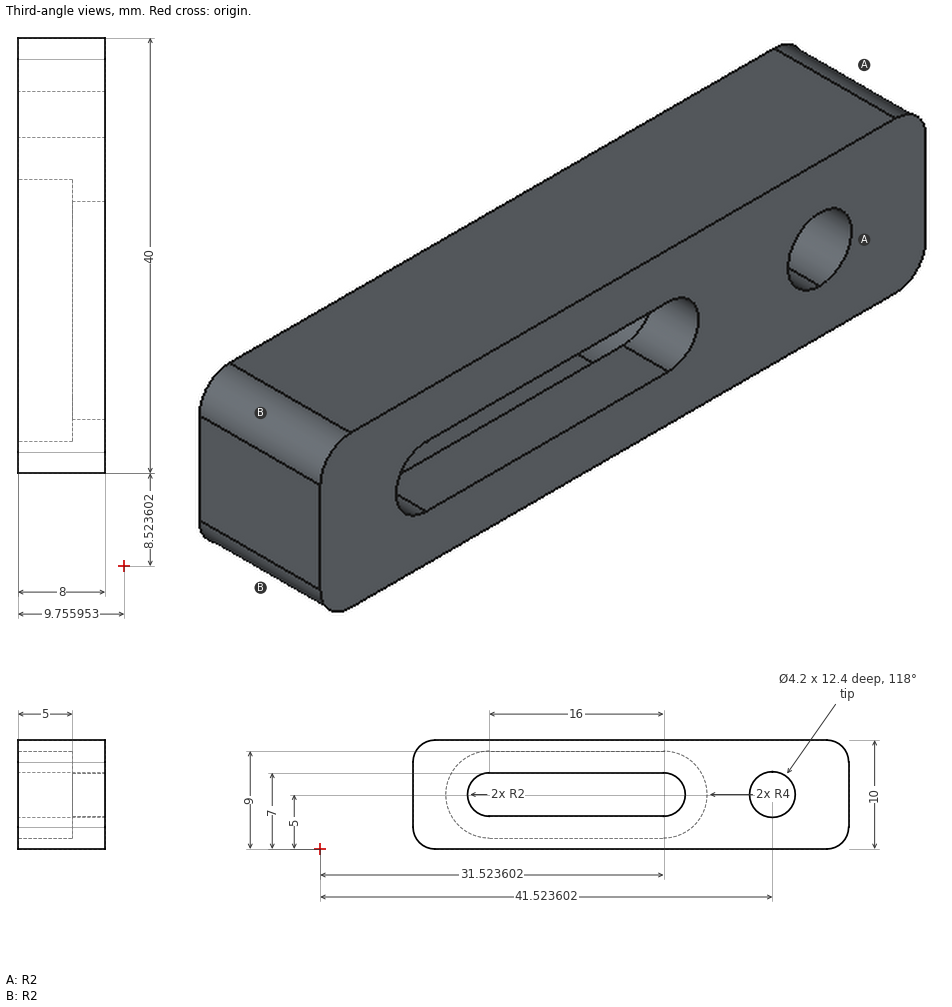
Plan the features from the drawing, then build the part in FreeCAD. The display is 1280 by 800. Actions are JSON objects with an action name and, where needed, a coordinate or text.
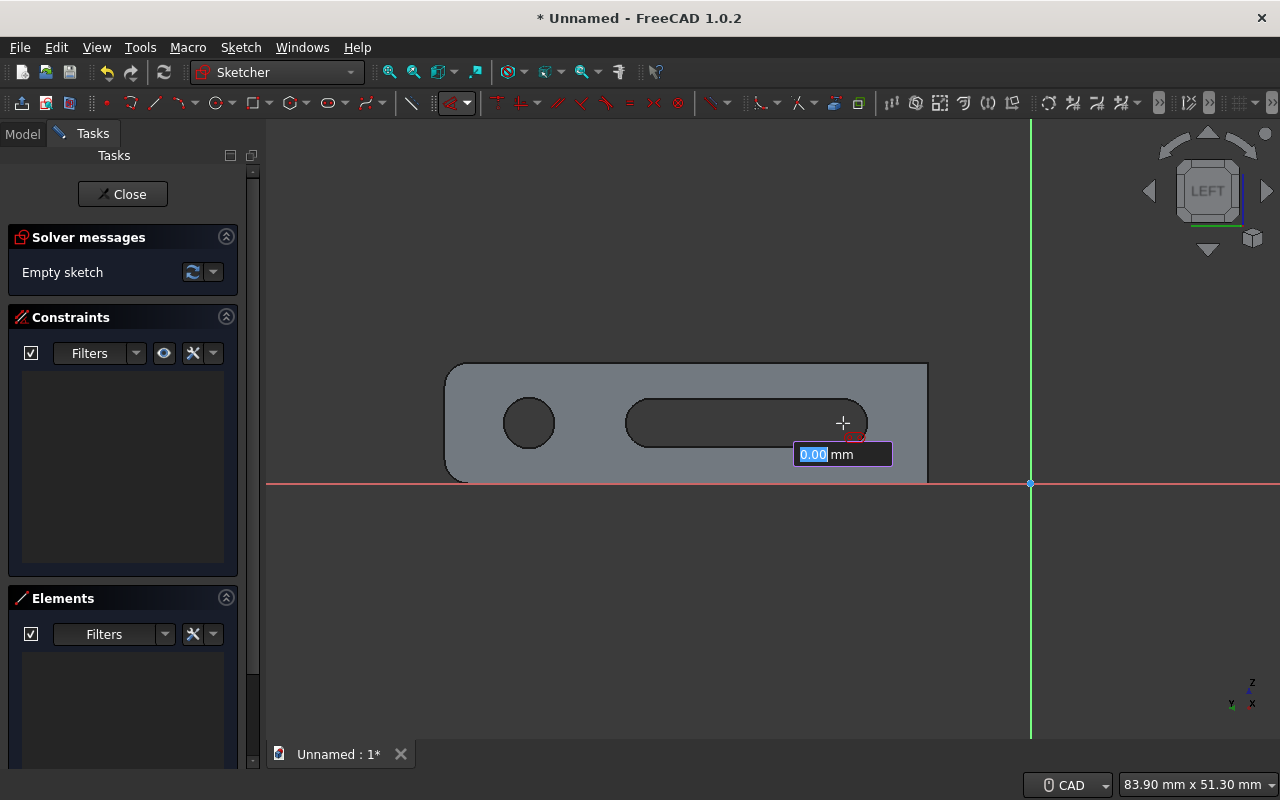
{"action": "left_click", "coordinate": [747, 375]}
{"action": "key", "text": "Escape"}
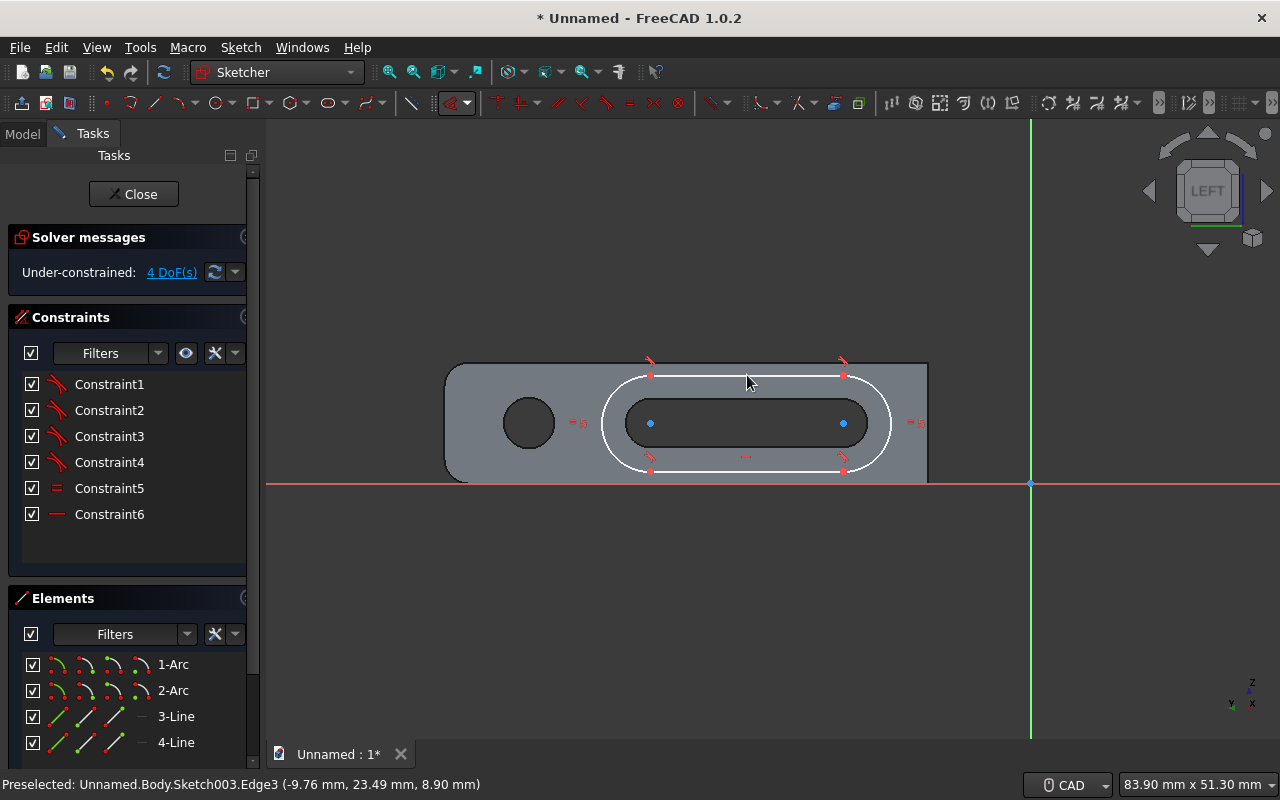
{"action": "key", "text": "d"}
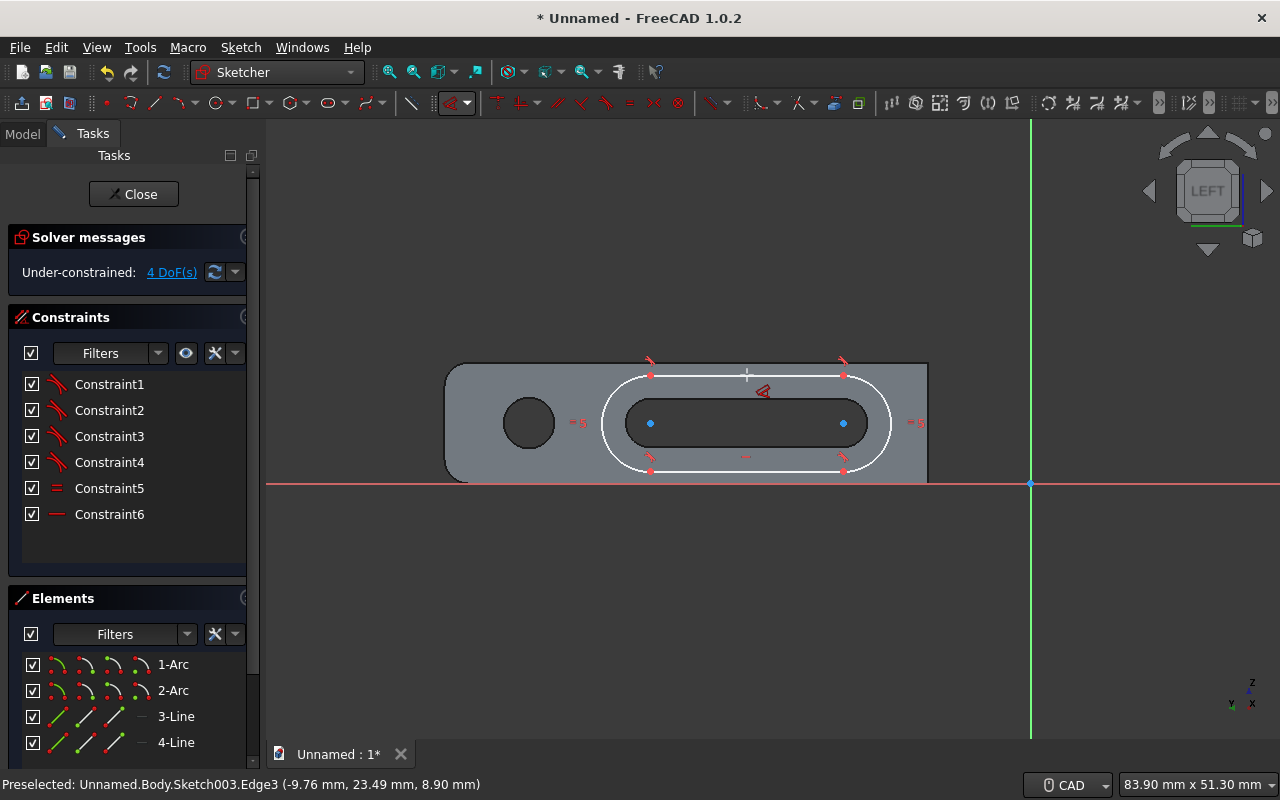
{"action": "left_click", "coordinate": [611, 396]}
{"action": "left_click", "coordinate": [585, 377]}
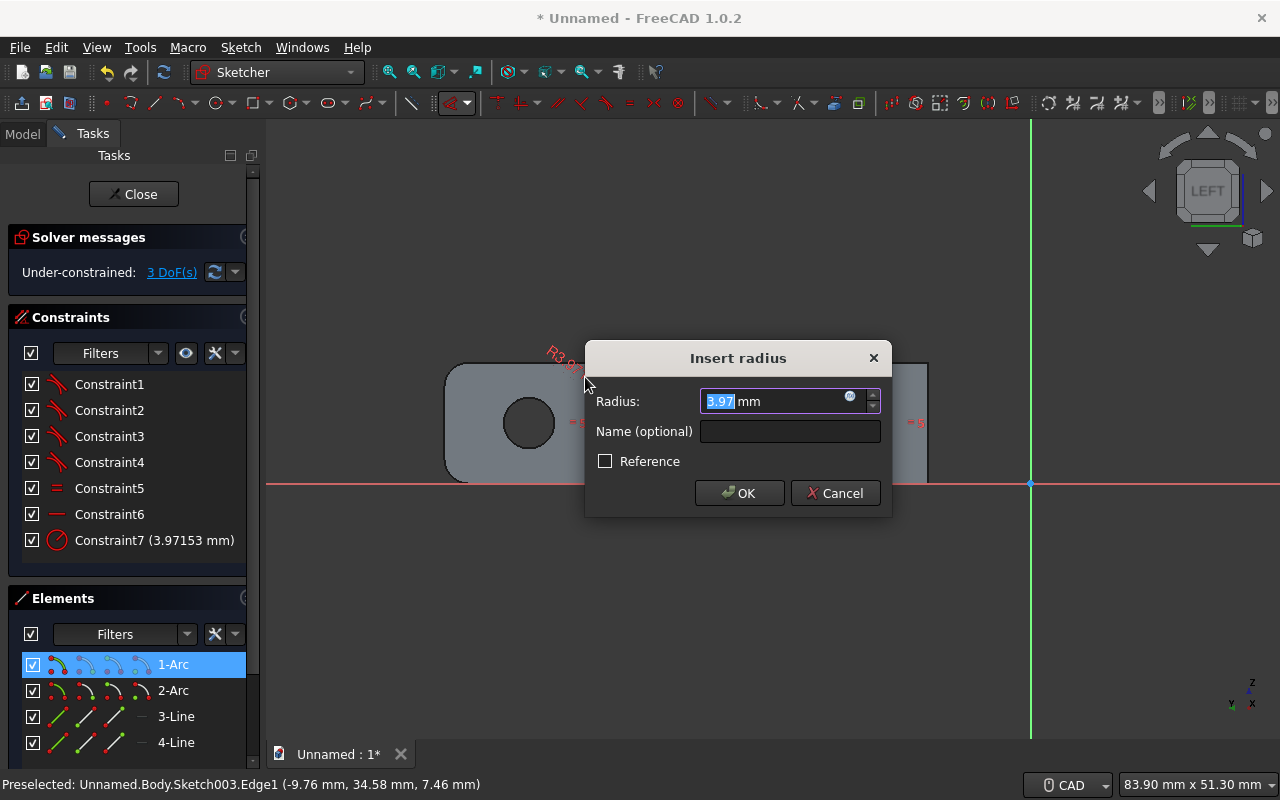
{"action": "type", "text": "4"}
{"action": "key", "text": "Return"}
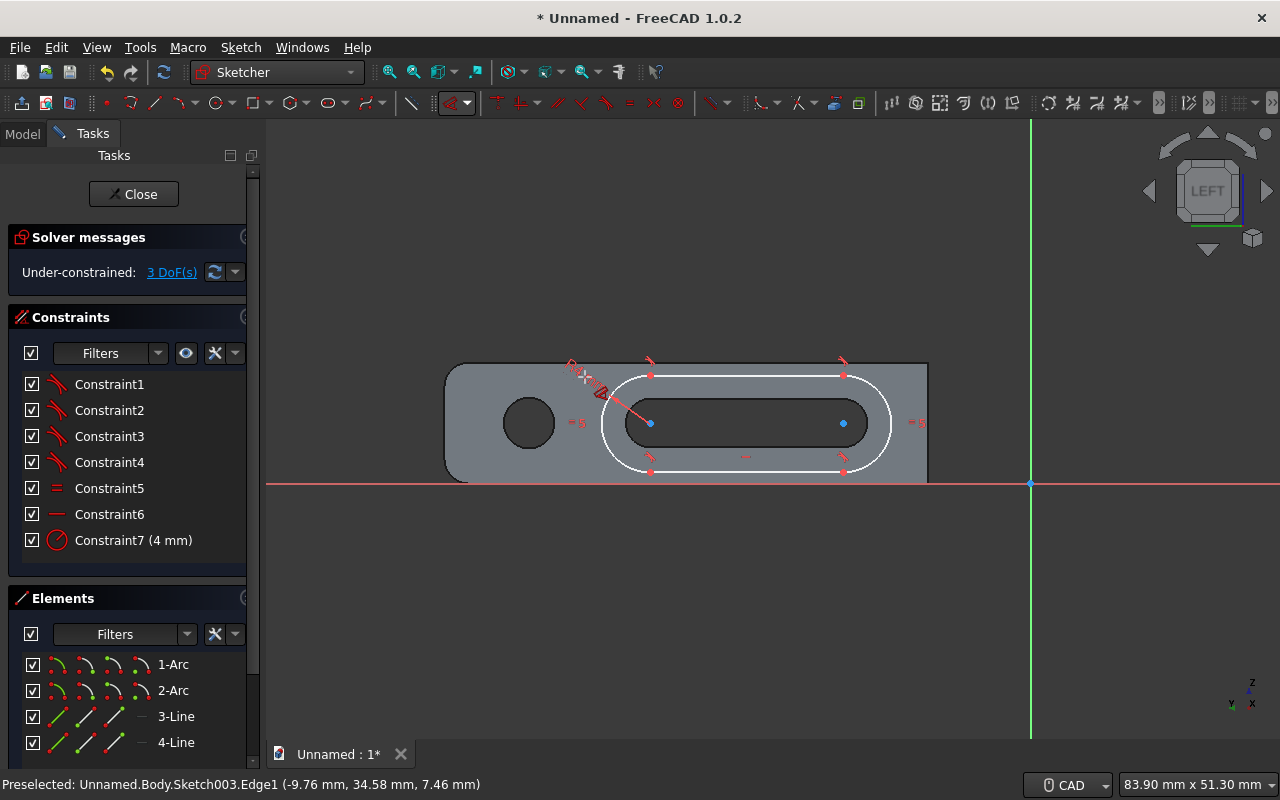
{"action": "left_click", "coordinate": [708, 376]}
{"action": "left_click", "coordinate": [746, 342]}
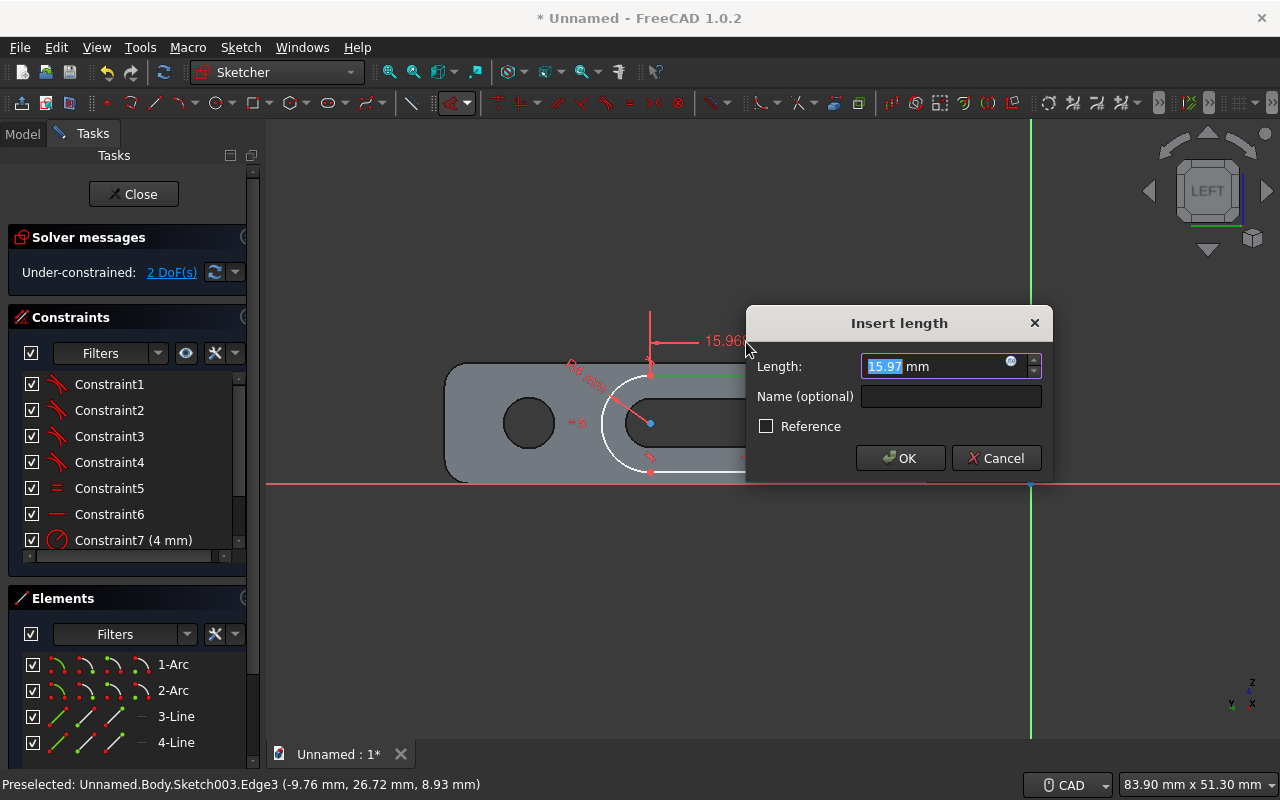
{"action": "type", "text": "16"}
{"action": "key", "text": "Return"}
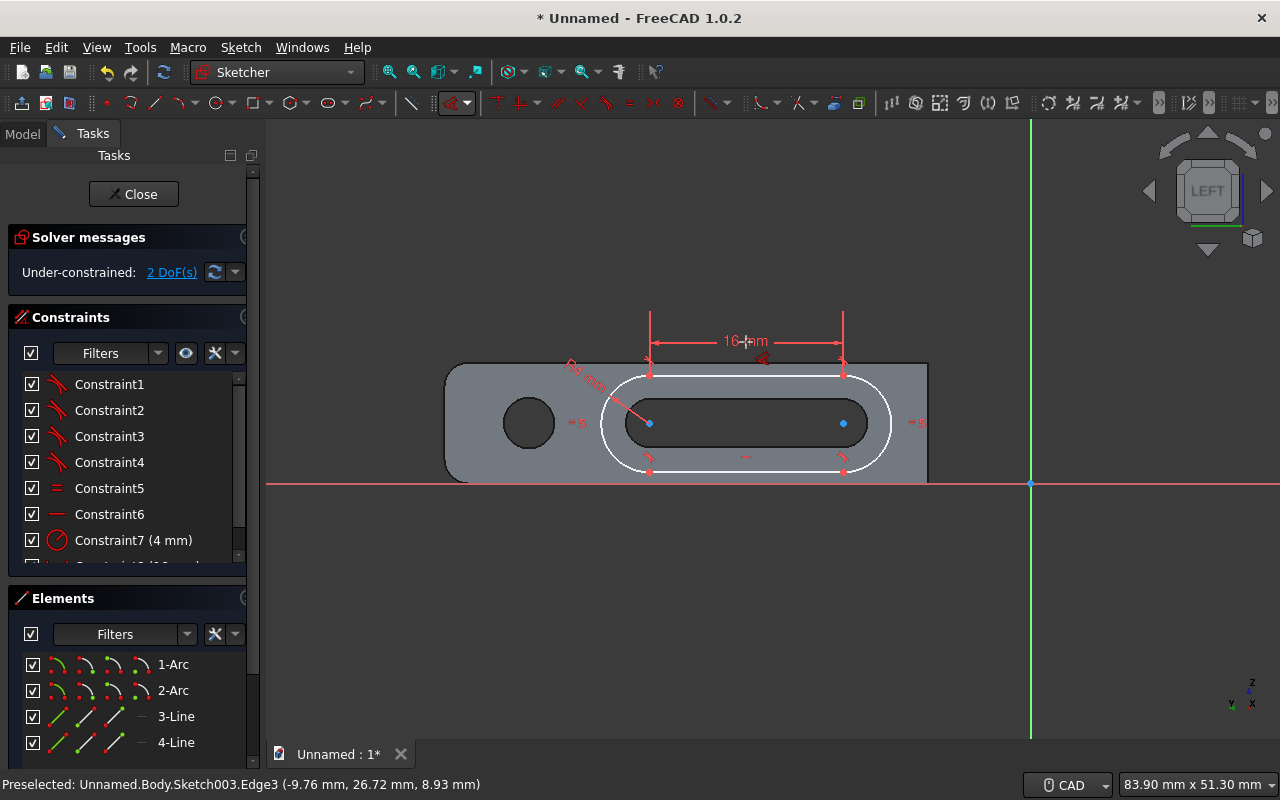
{"action": "left_click", "coordinate": [650, 376]}
{"action": "left_click", "coordinate": [1065, 430]}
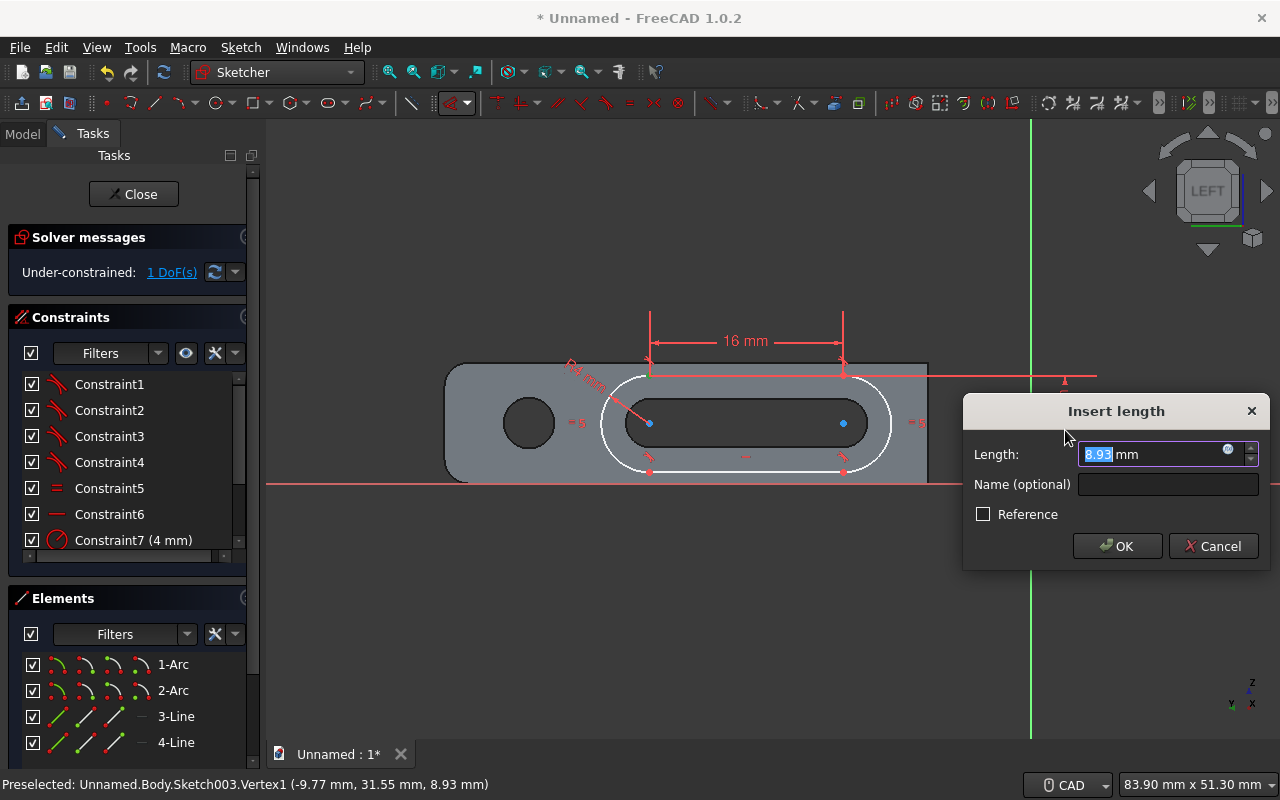
{"action": "type", "text": "9"}
{"action": "key", "text": "Return"}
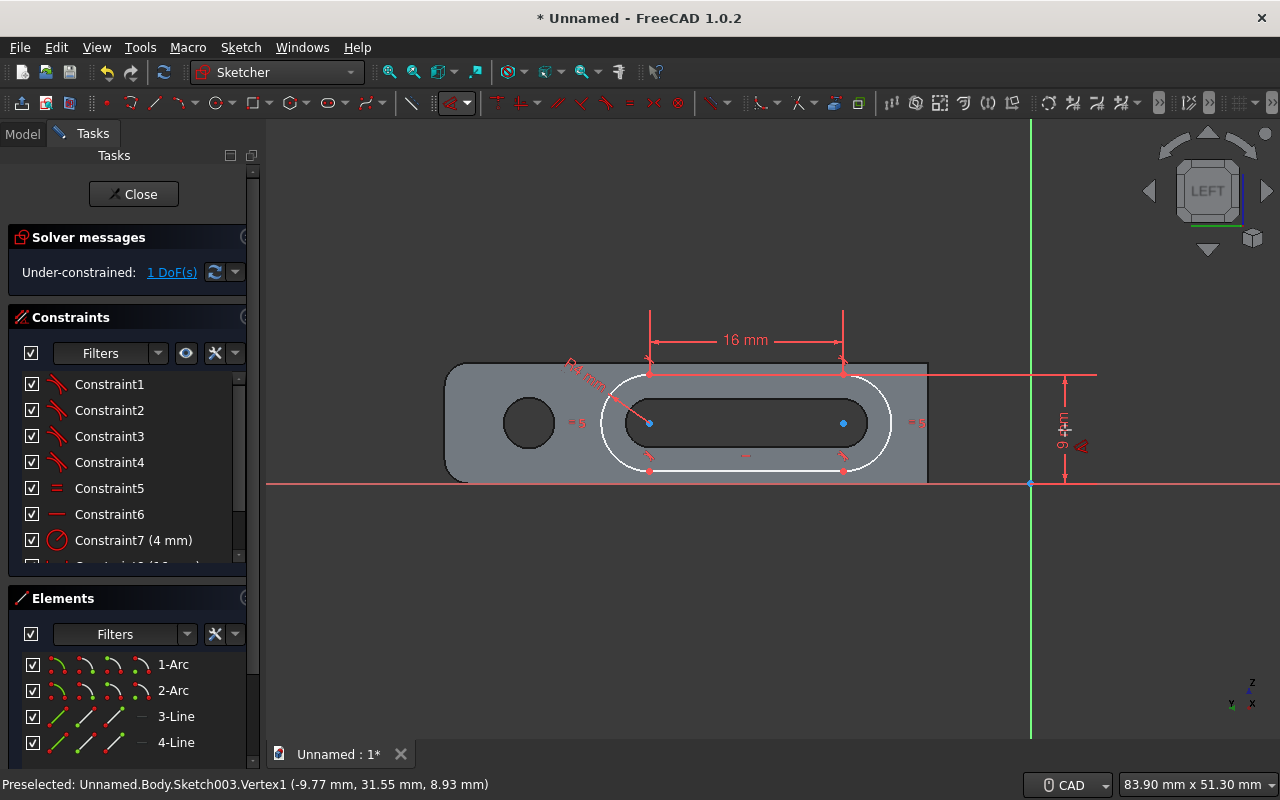
{"action": "left_click", "coordinate": [650, 375]}
{"action": "left_click", "coordinate": [840, 518]}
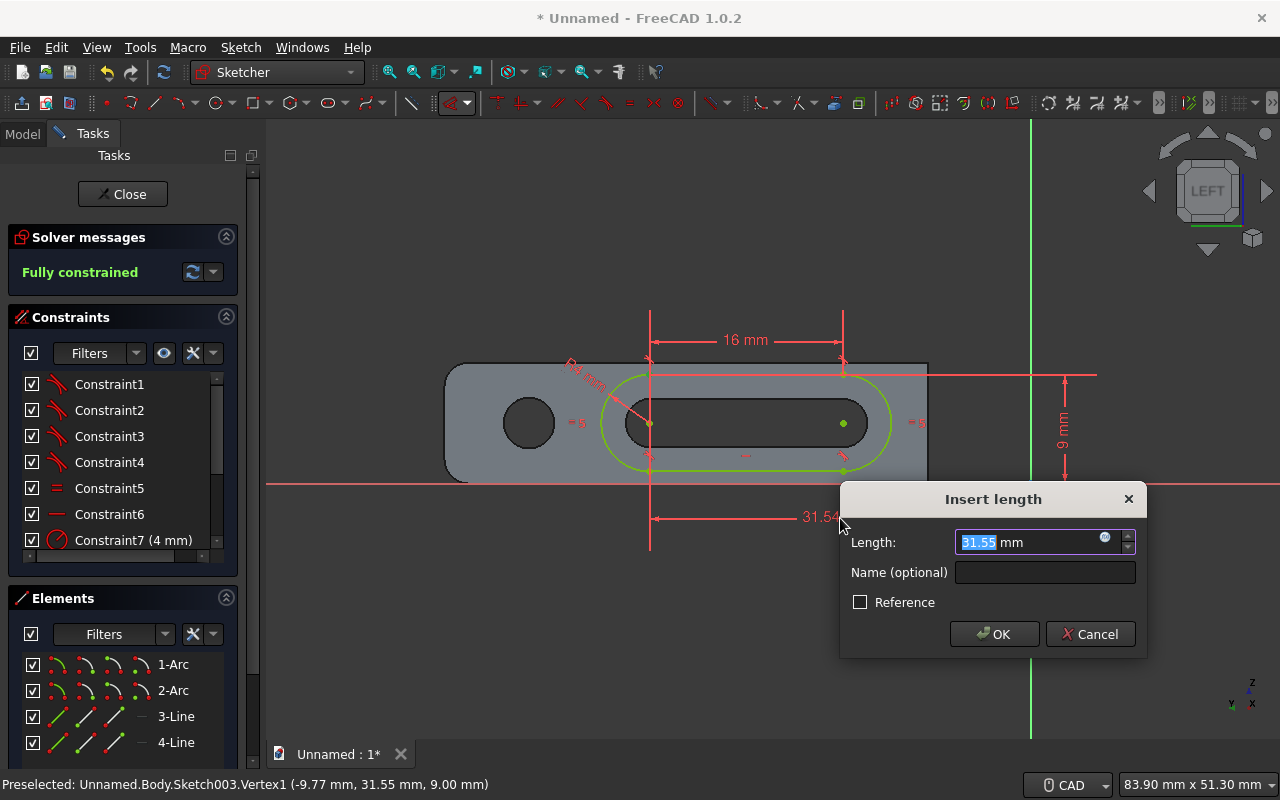
{"action": "type", "text": "31.523602"}
{"action": "key", "text": "Return"}
{"action": "key", "text": "Escape"}